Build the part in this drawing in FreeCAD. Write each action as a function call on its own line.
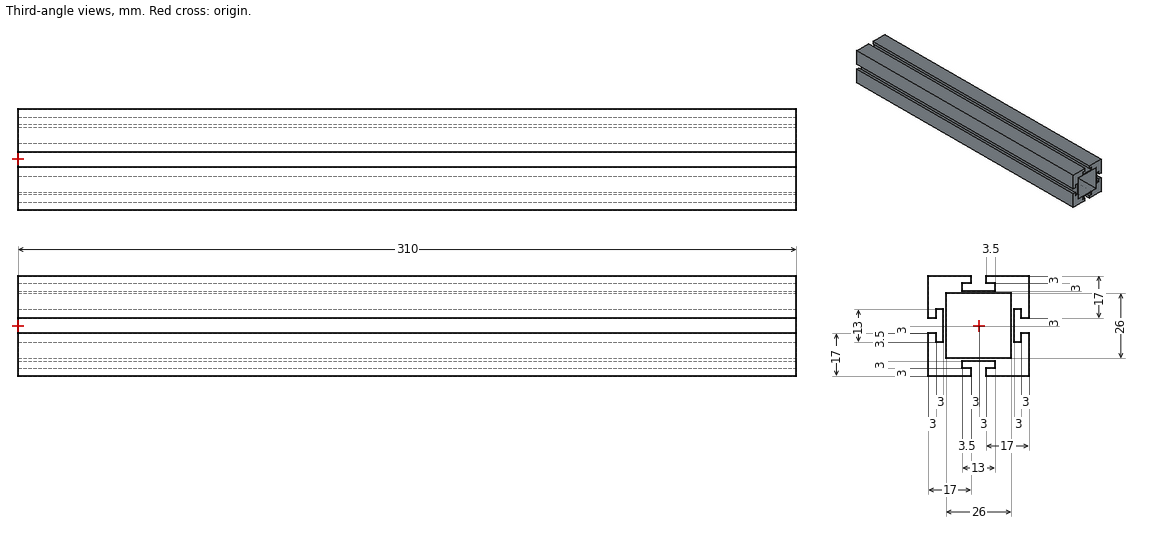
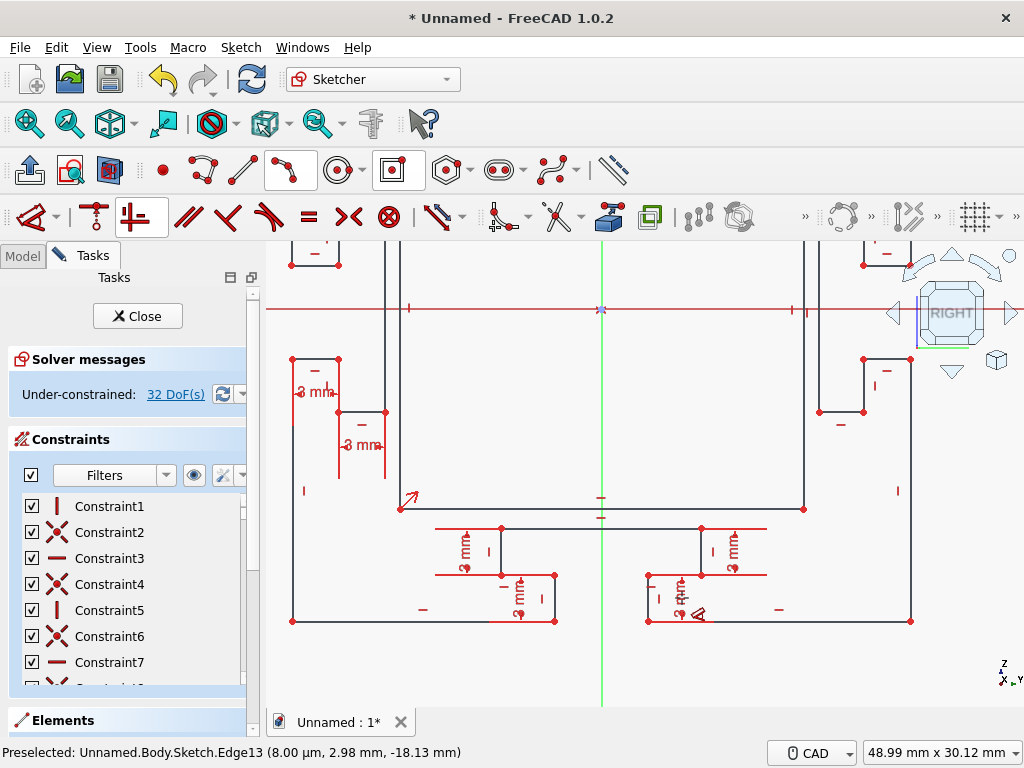
scroll(556, 608, down, 4)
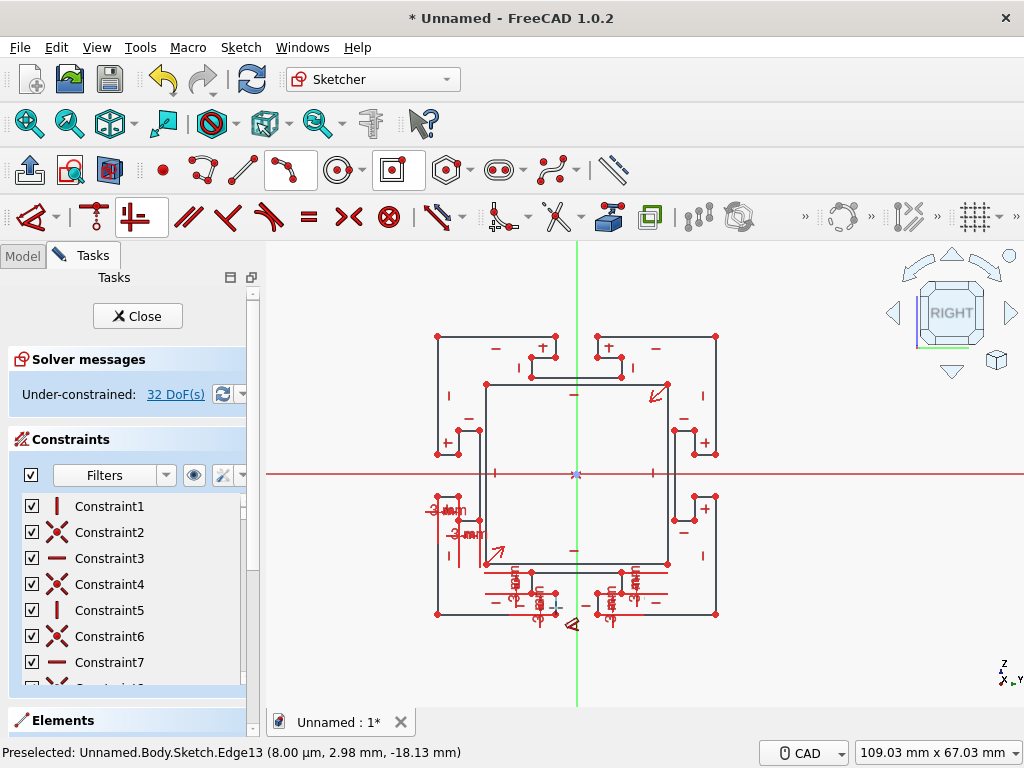
scroll(709, 497, up, 4)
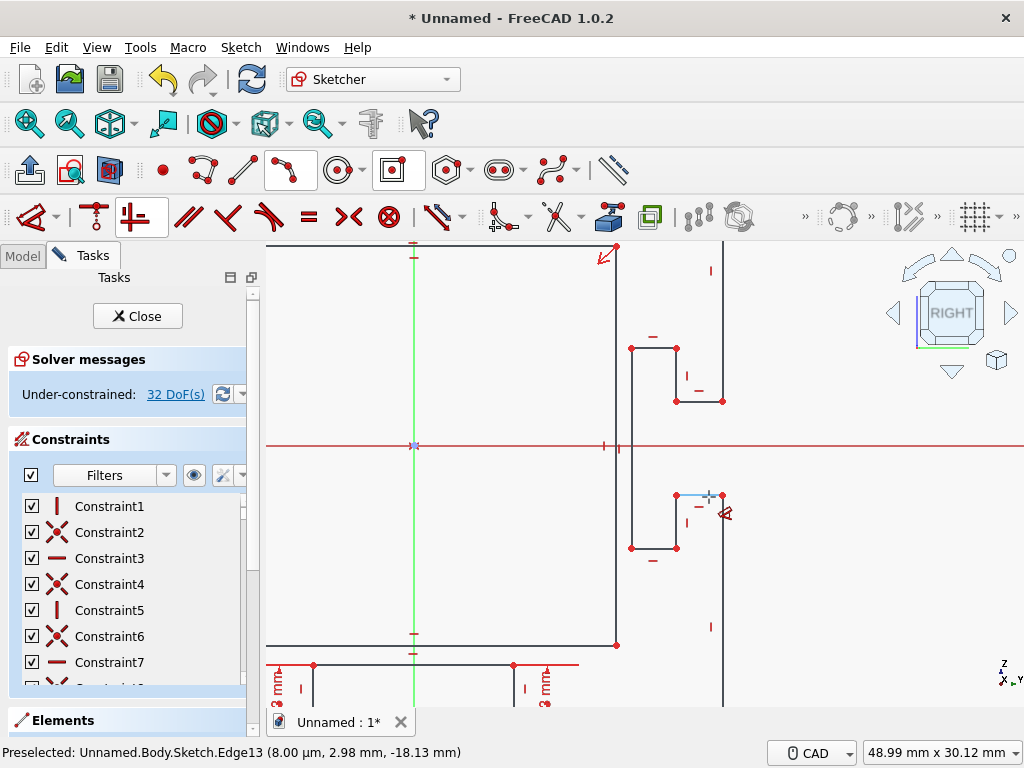
click(709, 495)
click(699, 529)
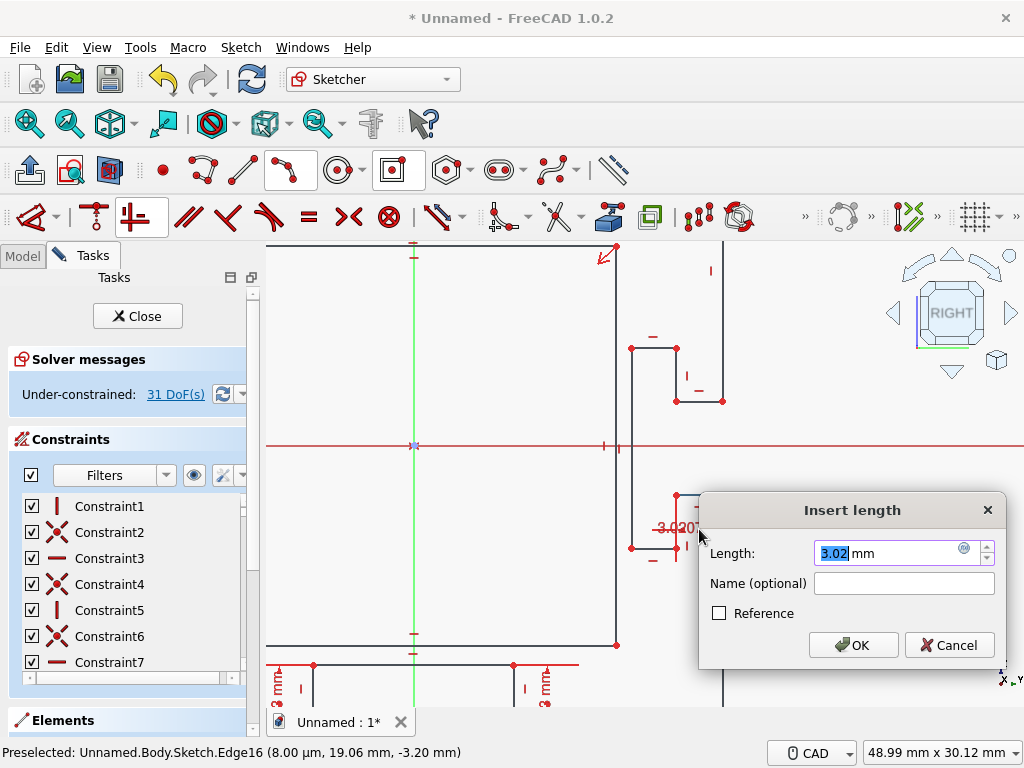
text(3)
key(Return)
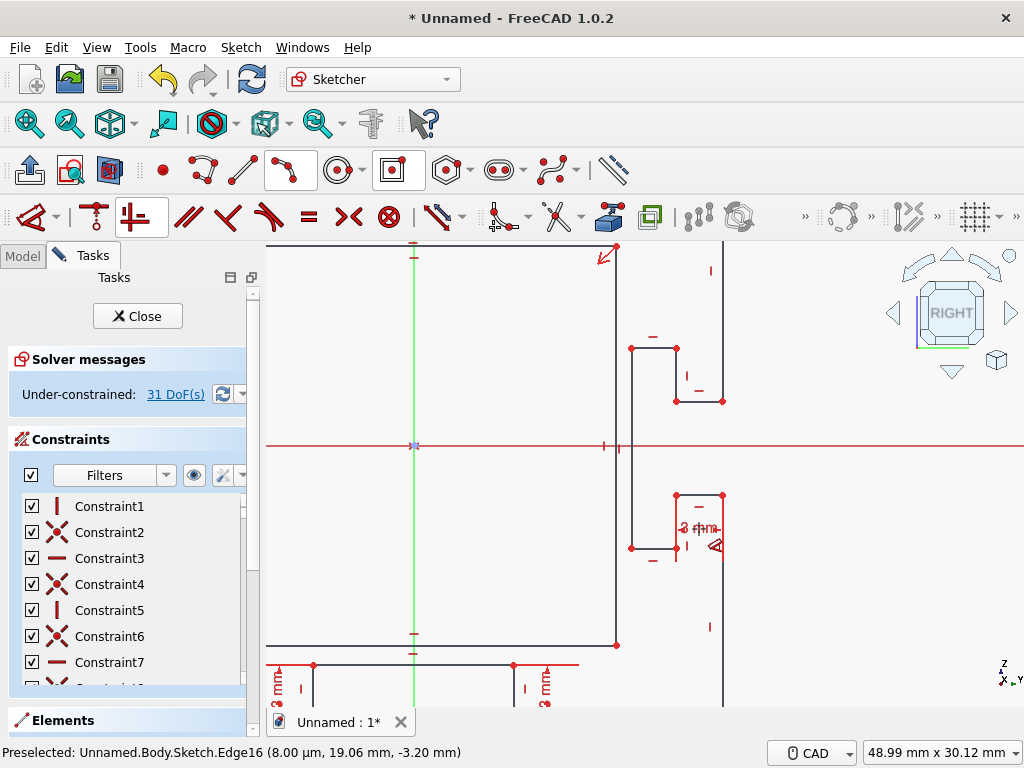
click(663, 549)
click(654, 583)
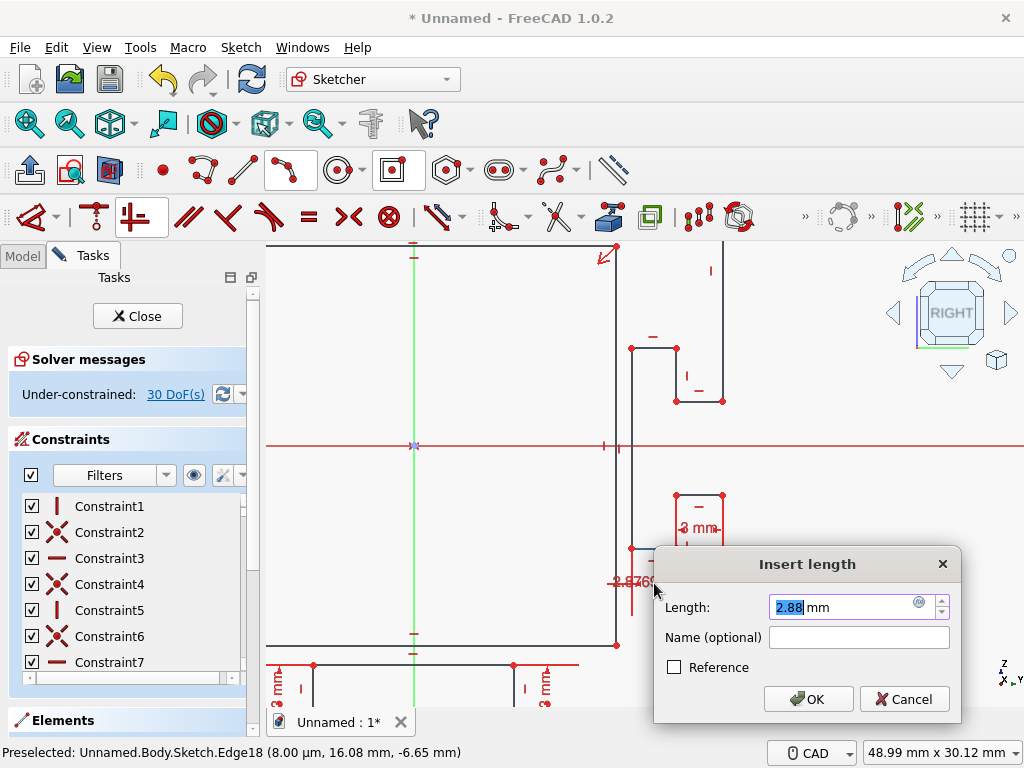
text(3)
key(Return)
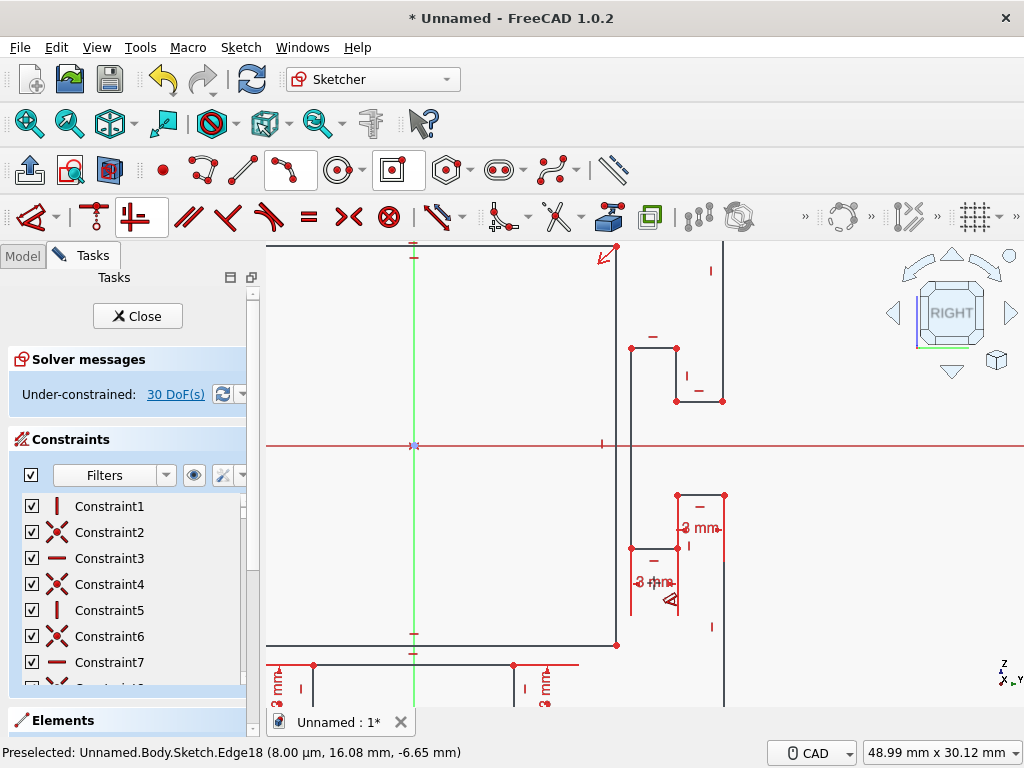
click(645, 348)
click(654, 314)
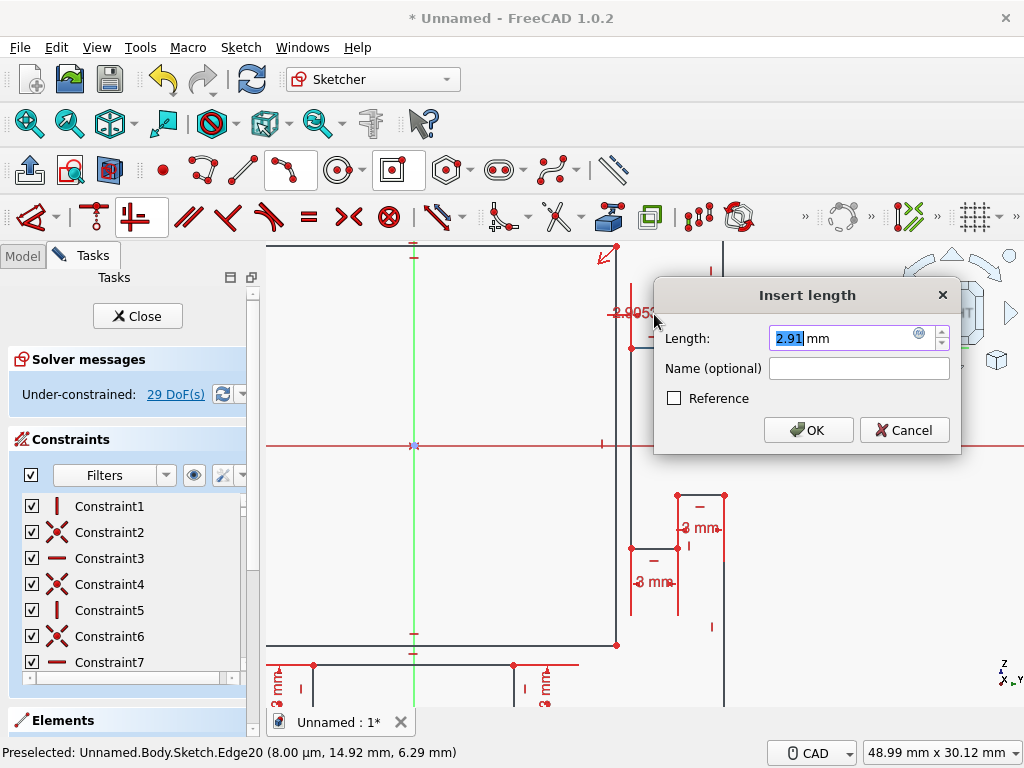
text(3)
key(Return)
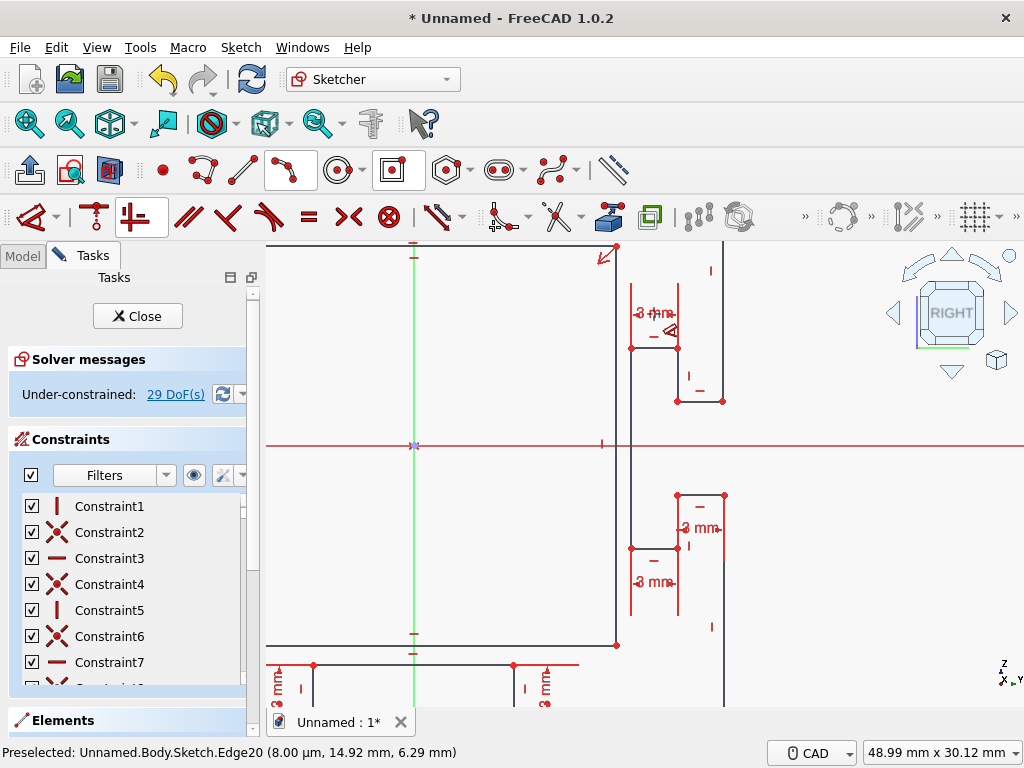
click(691, 402)
click(700, 368)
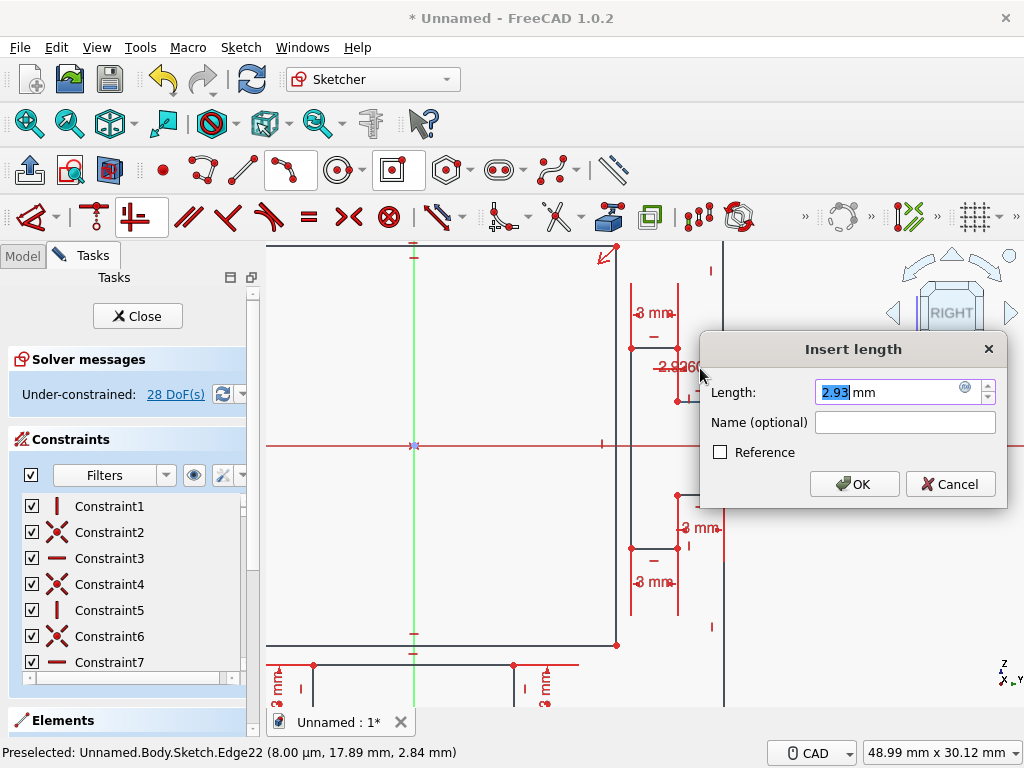
text(3)
key(Return)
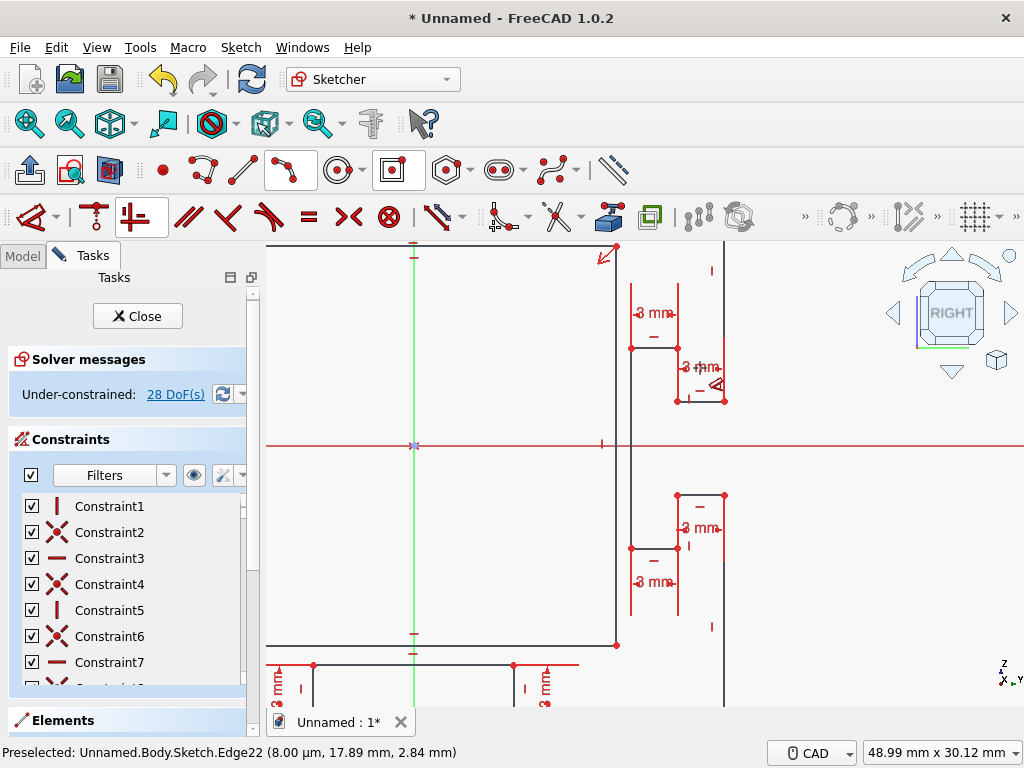
scroll(709, 497, down, 4)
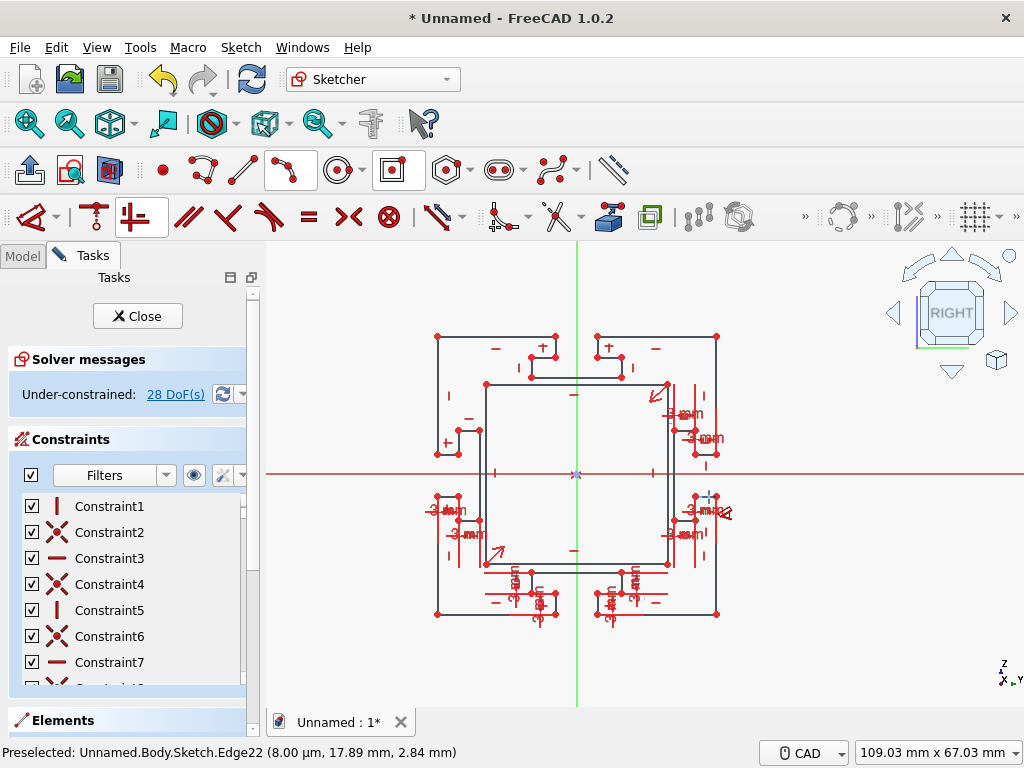
scroll(598, 343, up, 4)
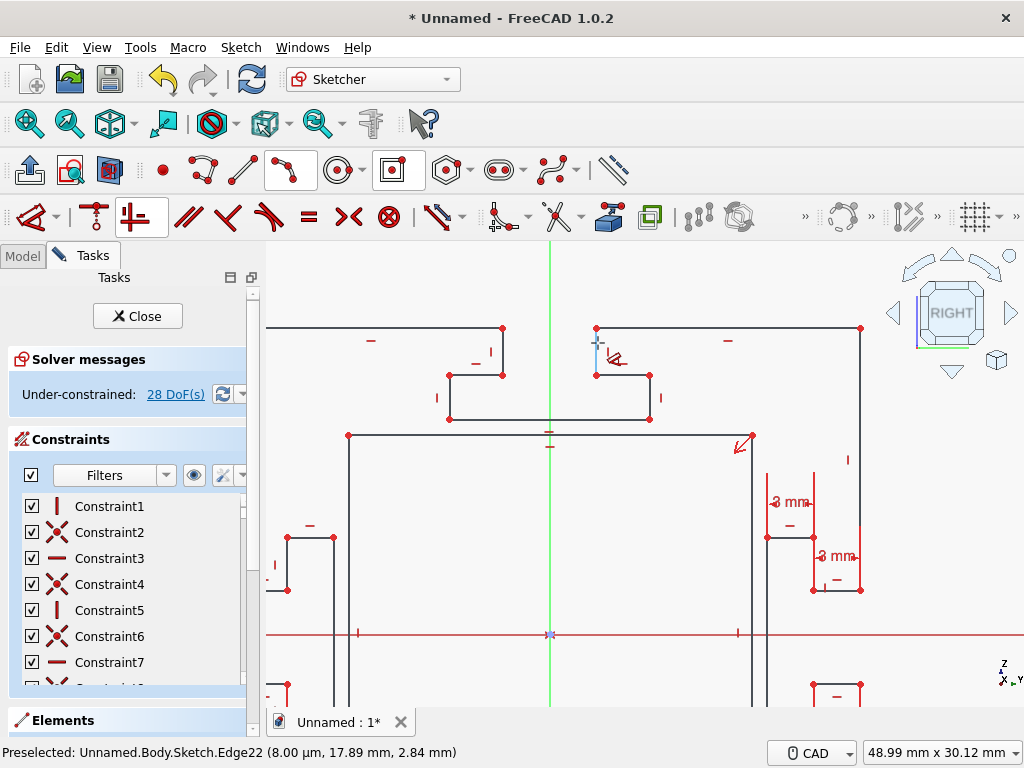
click(596, 342)
click(630, 352)